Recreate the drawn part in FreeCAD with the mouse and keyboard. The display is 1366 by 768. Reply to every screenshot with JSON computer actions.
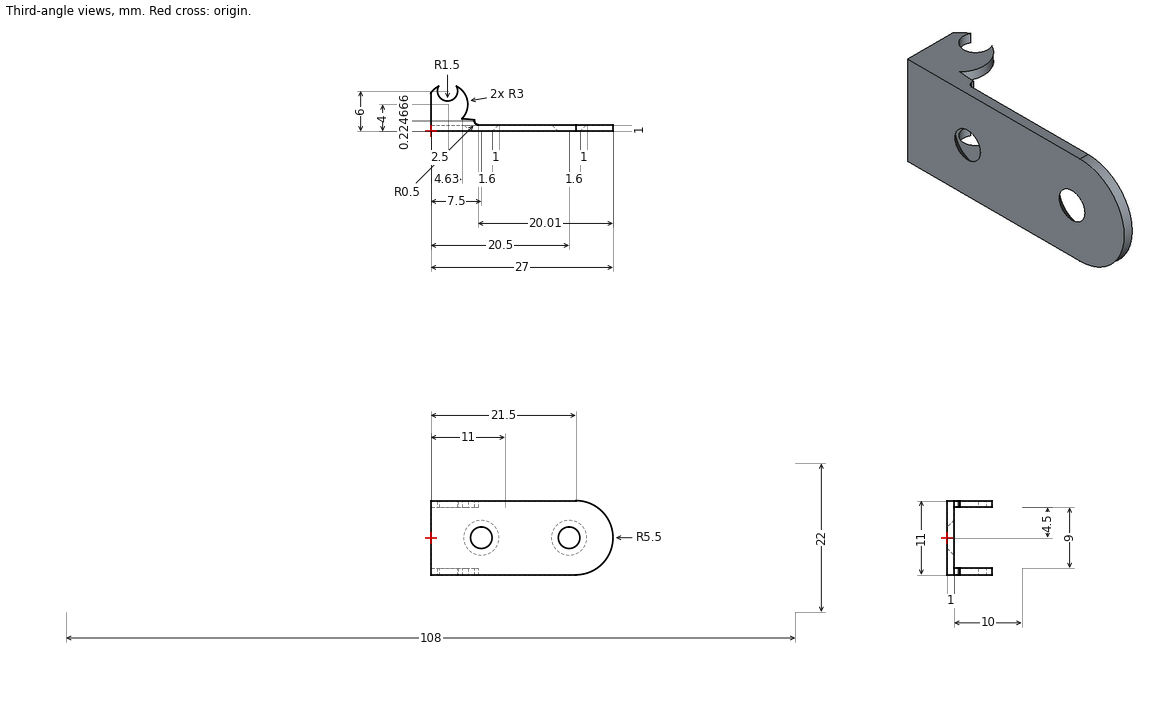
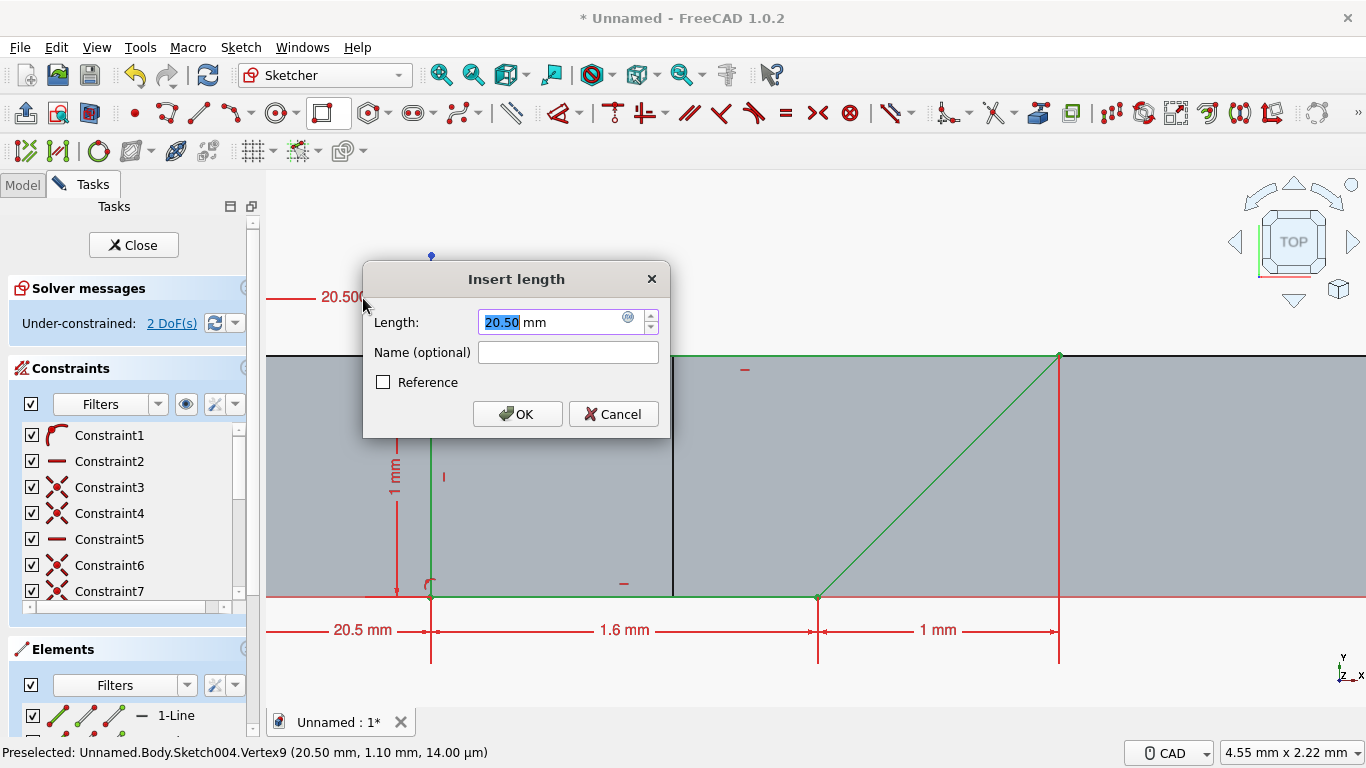
{"action": "type", "text": "20.5"}
{"action": "key", "text": "Return"}
{"action": "key", "text": "Escape"}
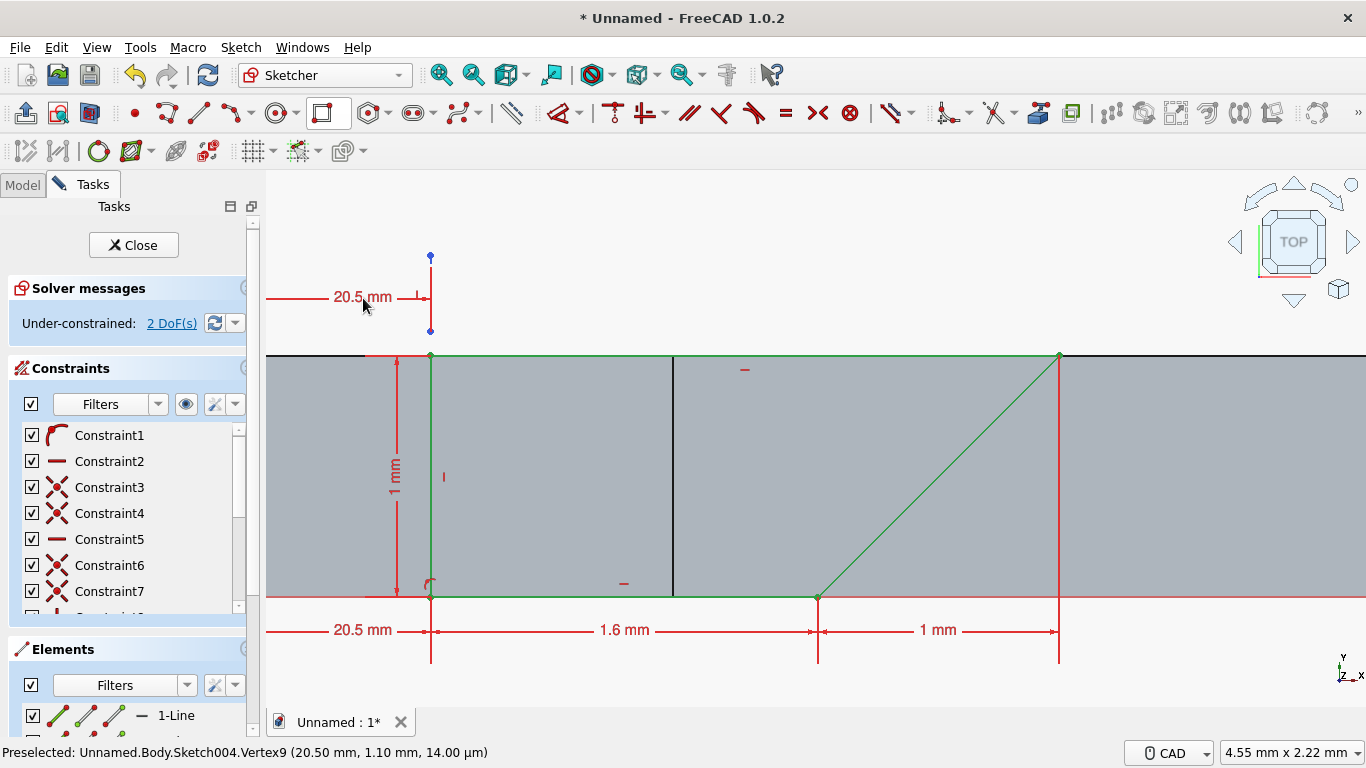
{"action": "left_click", "coordinate": [134, 245]}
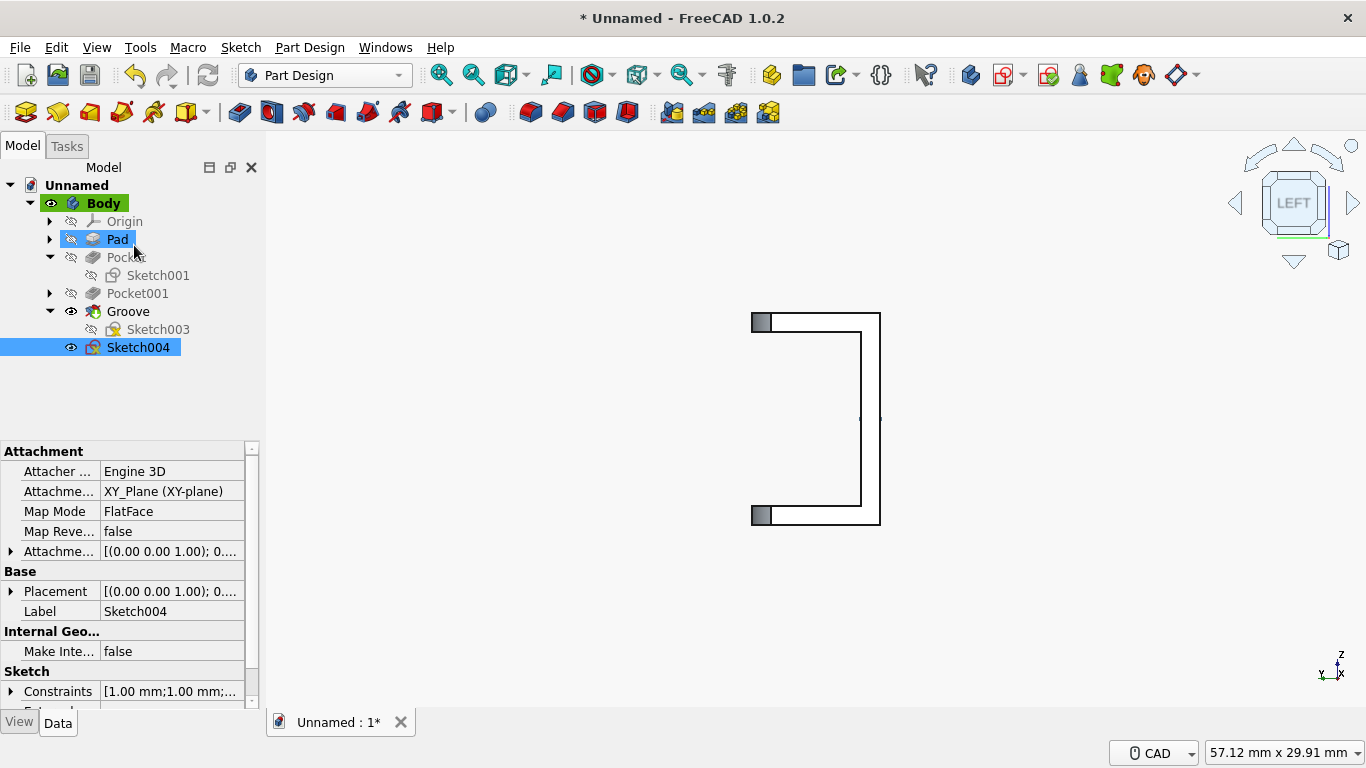
{"action": "left_click", "coordinate": [304, 112]}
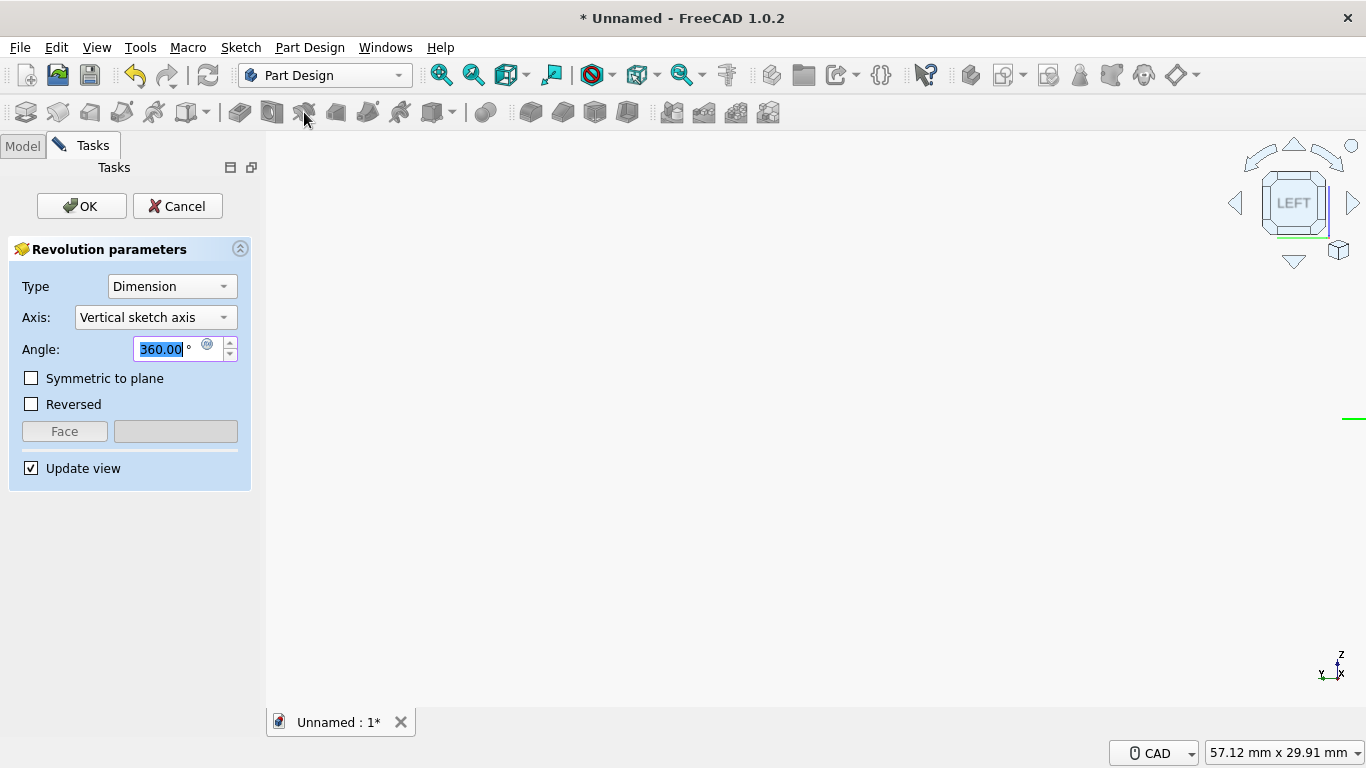
{"action": "left_click", "coordinate": [156, 318]}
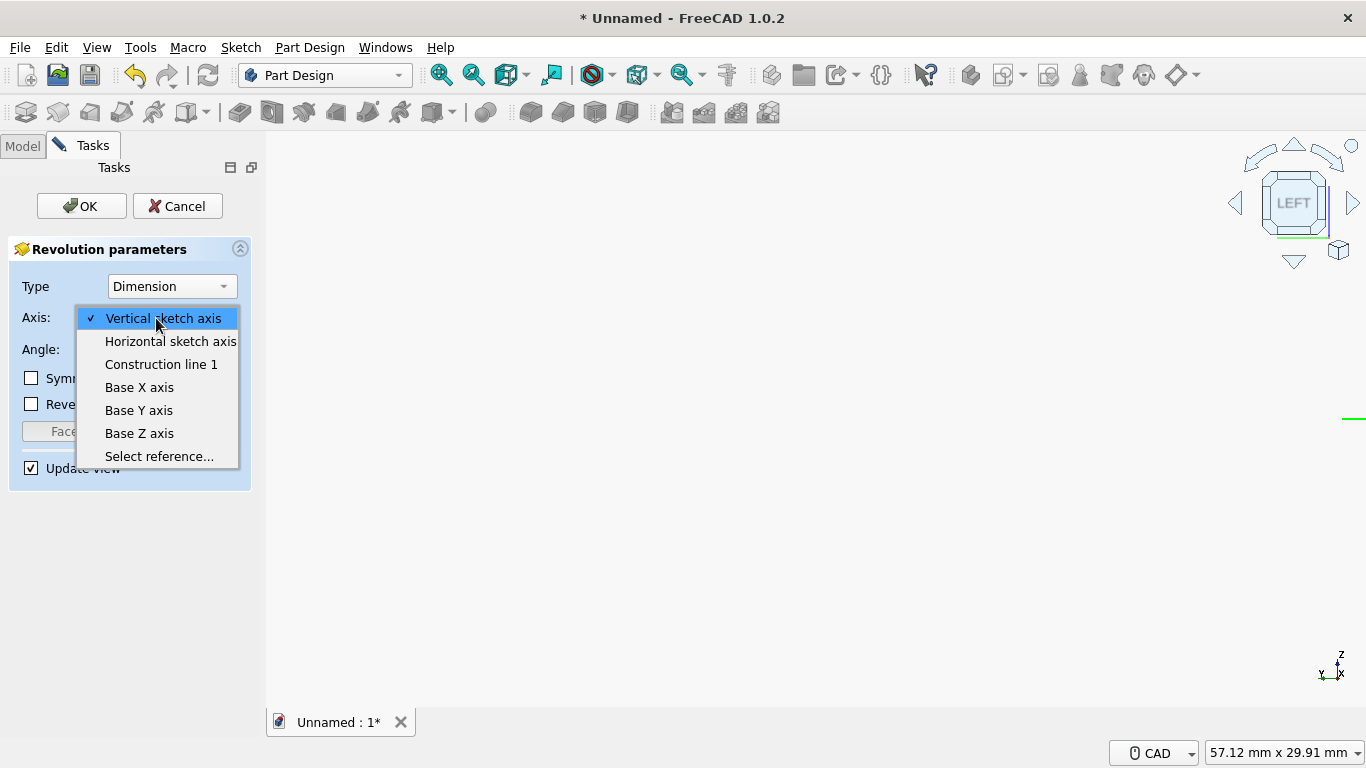
{"action": "left_click", "coordinate": [156, 364]}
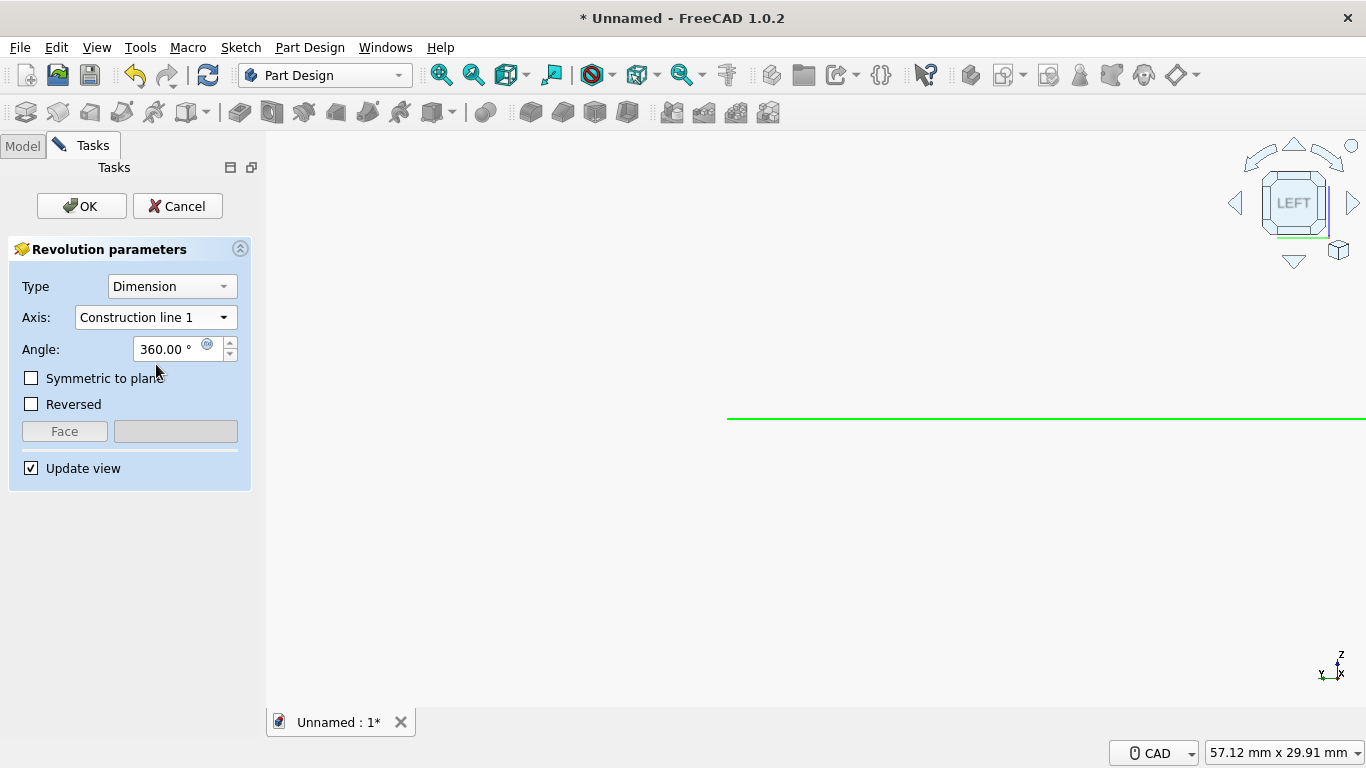
{"action": "left_click", "coordinate": [82, 206]}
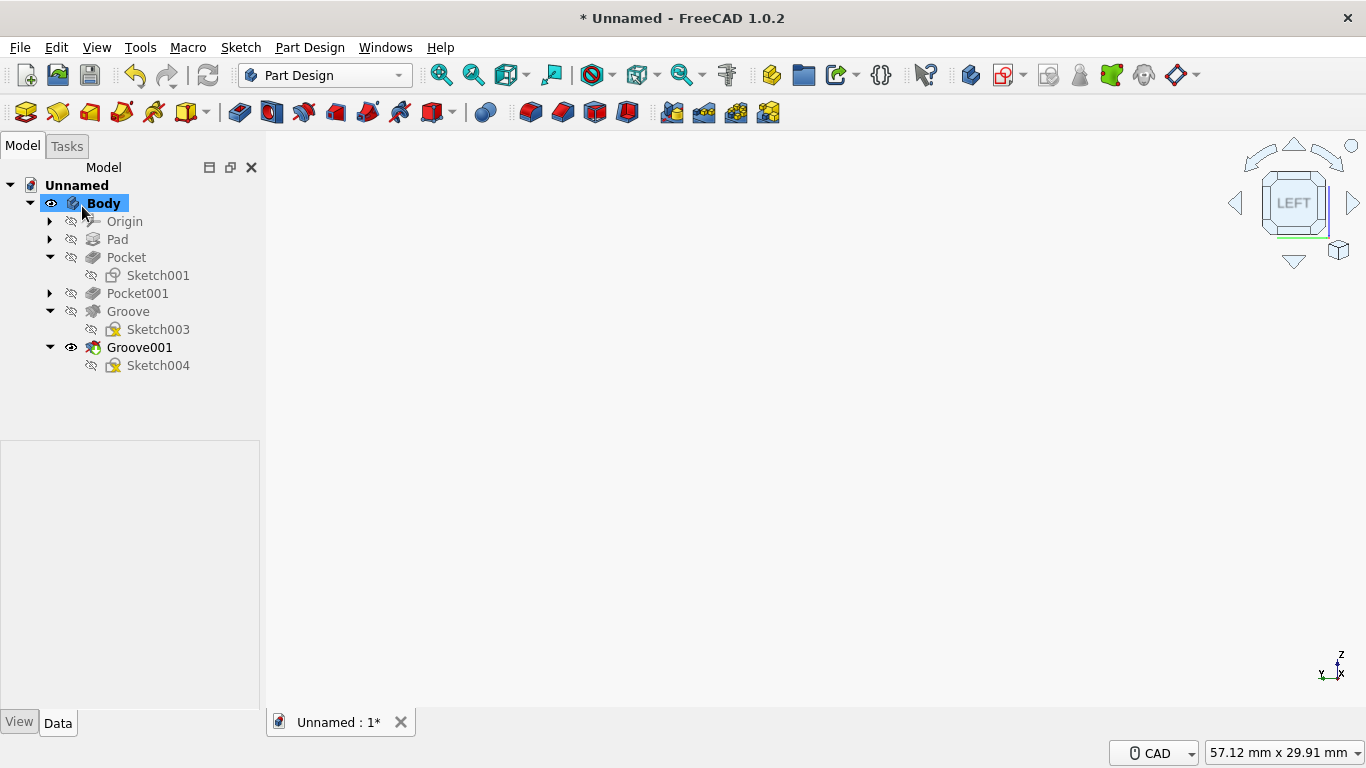
{"action": "key", "text": "0"}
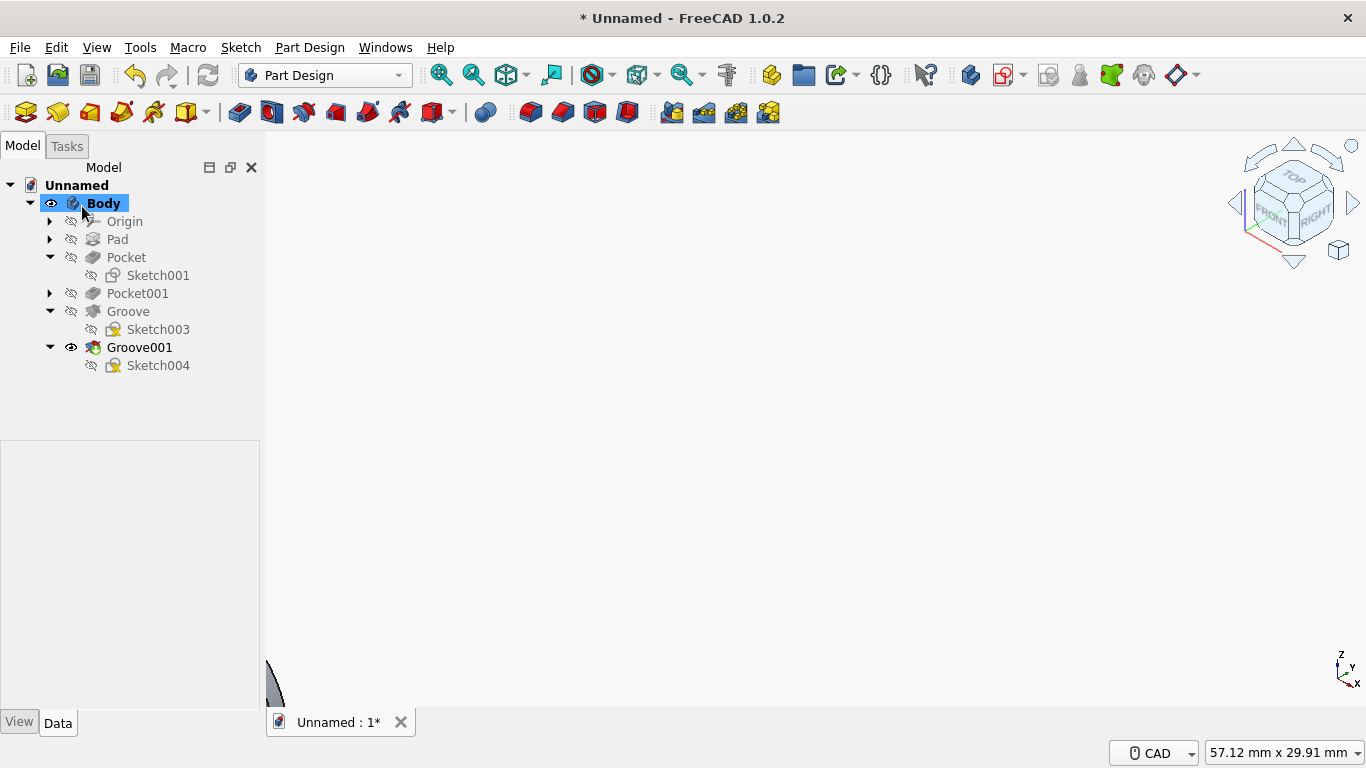
{"action": "left_click", "coordinate": [442, 76]}